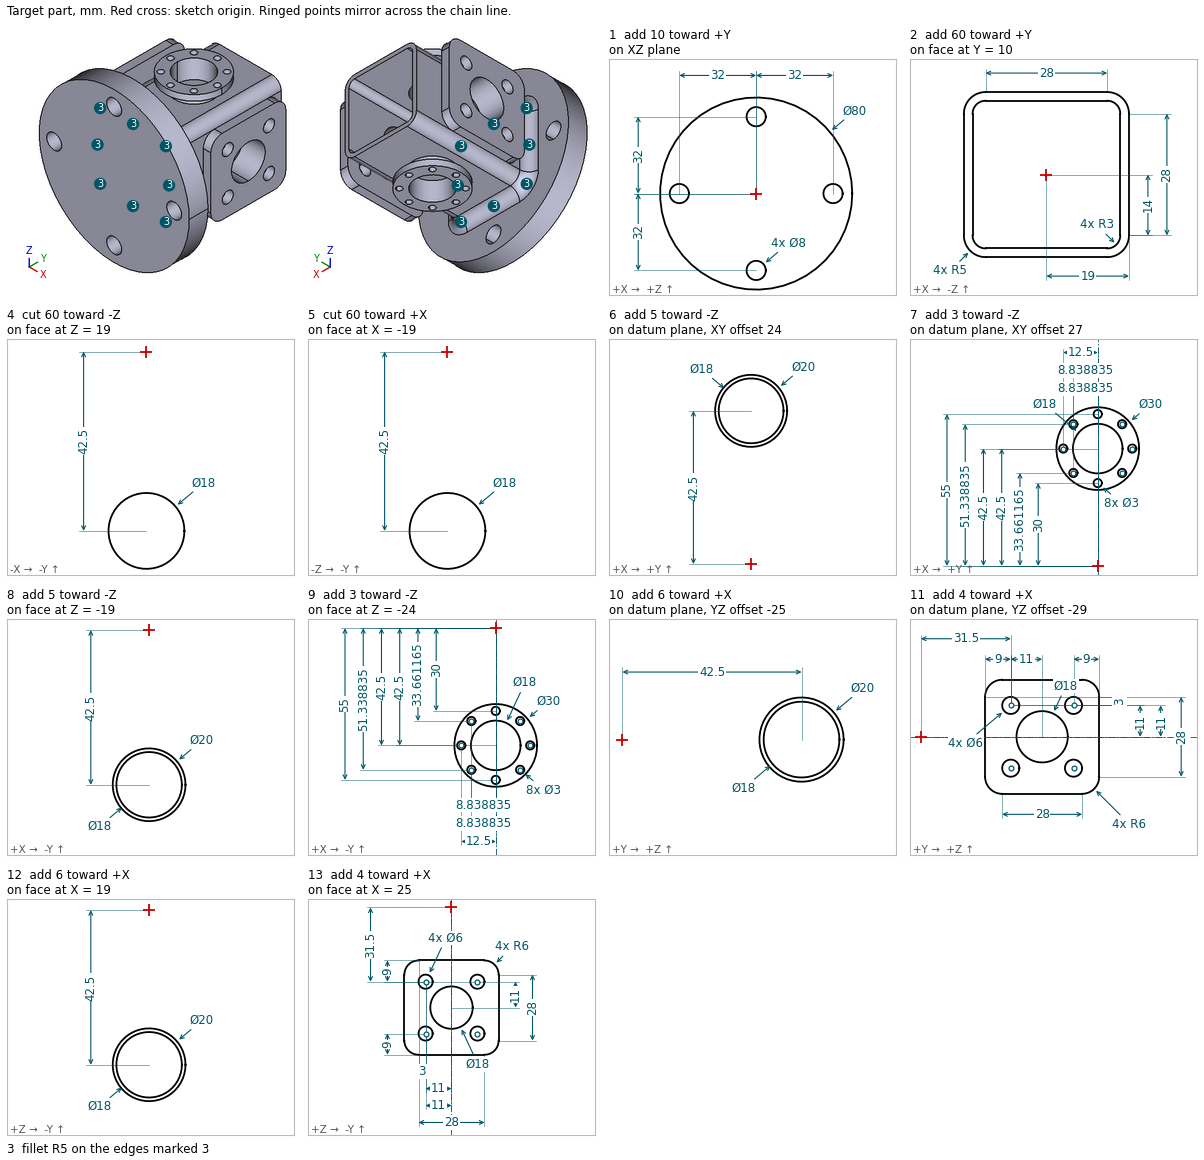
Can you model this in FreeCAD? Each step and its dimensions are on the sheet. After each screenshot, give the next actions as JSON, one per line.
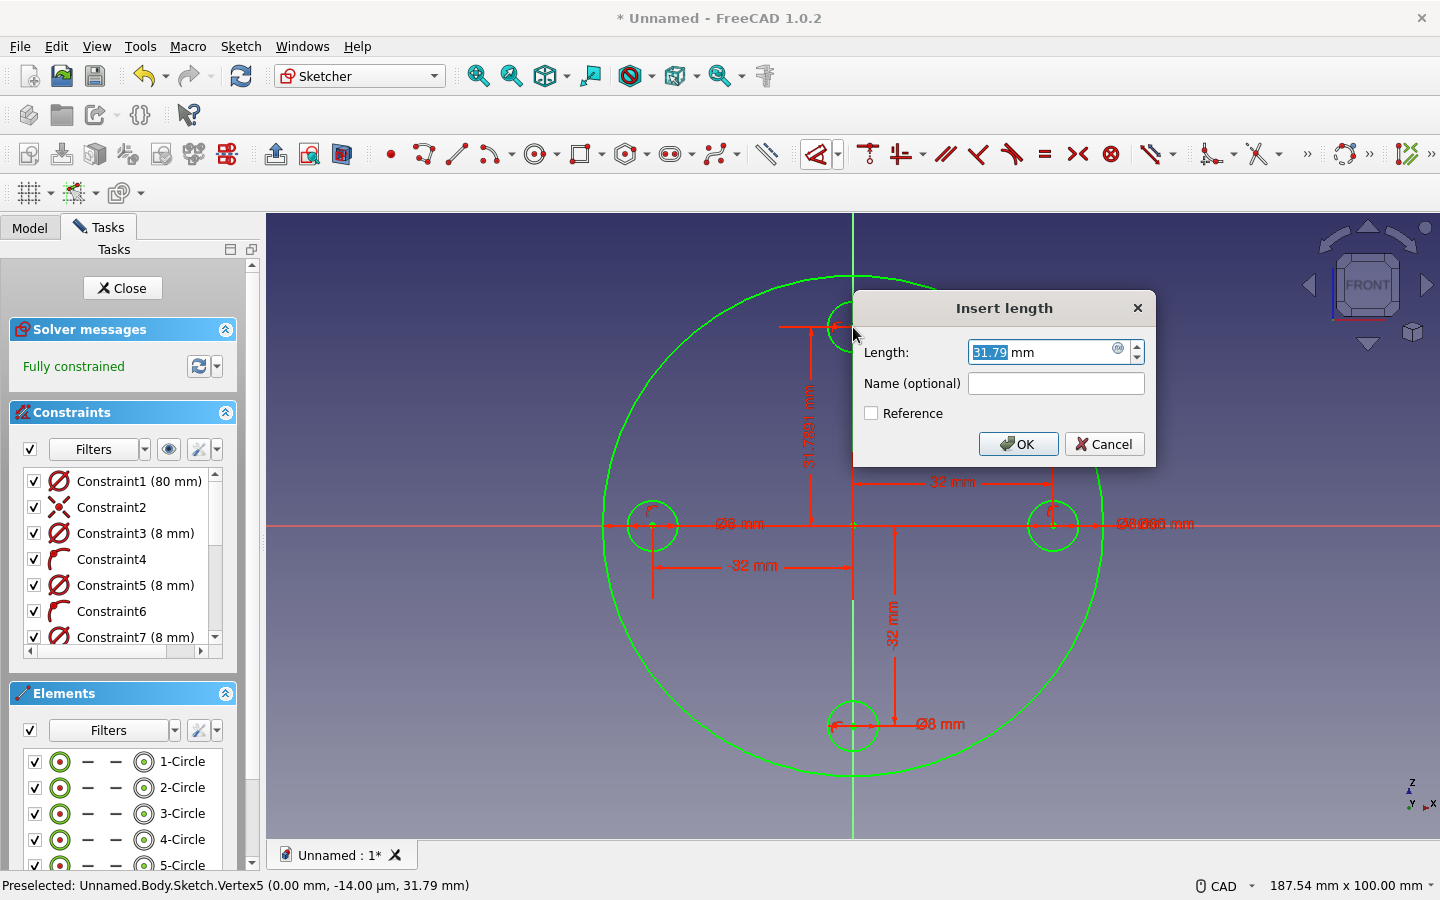
{"action": "type", "text": "32"}
{"action": "key", "text": "Return"}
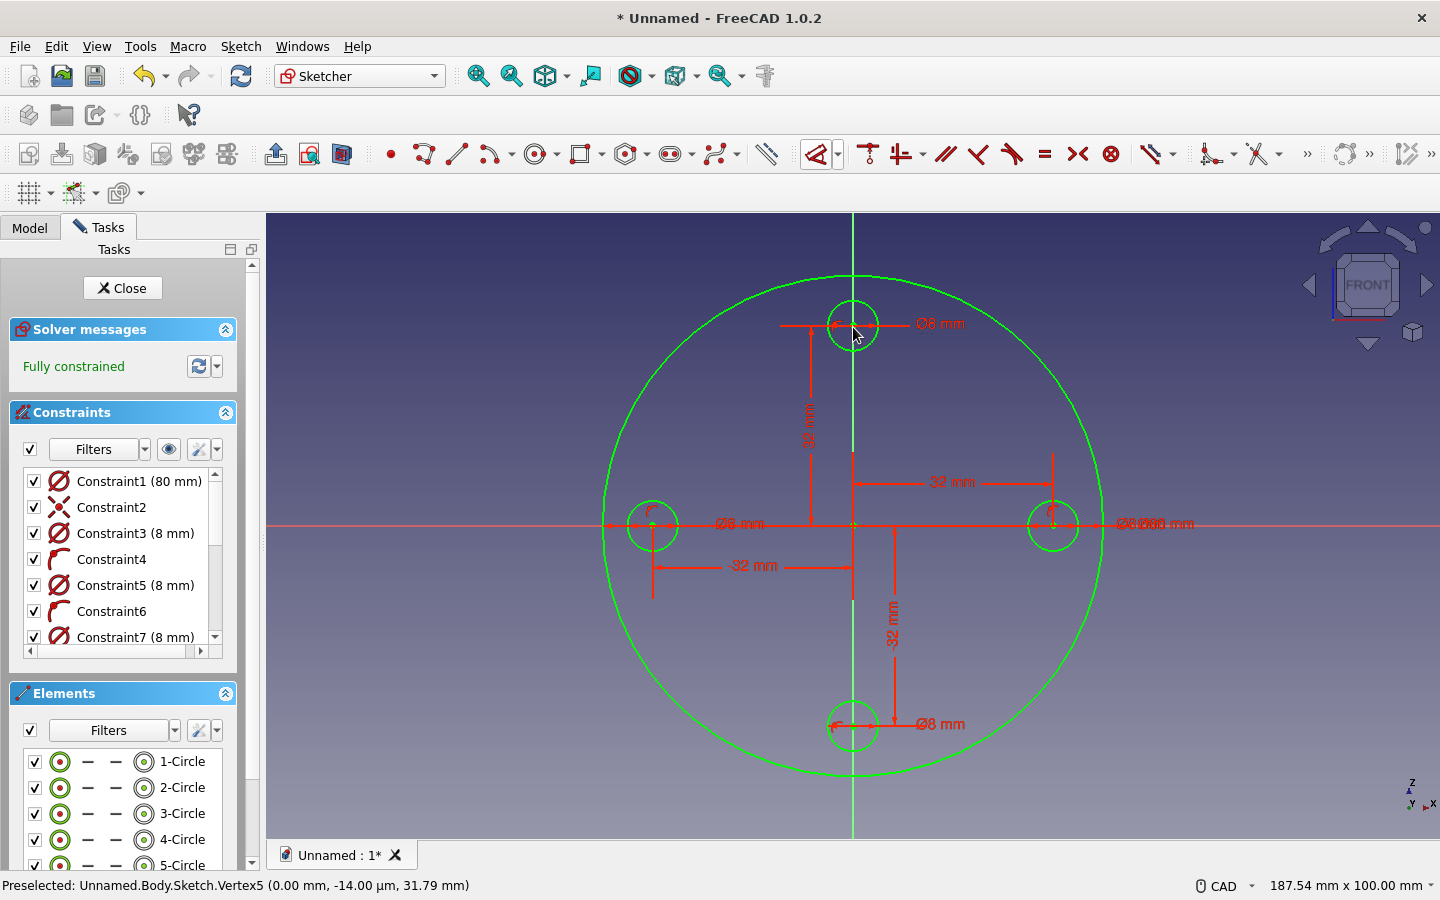
{"action": "left_click", "coordinate": [123, 288]}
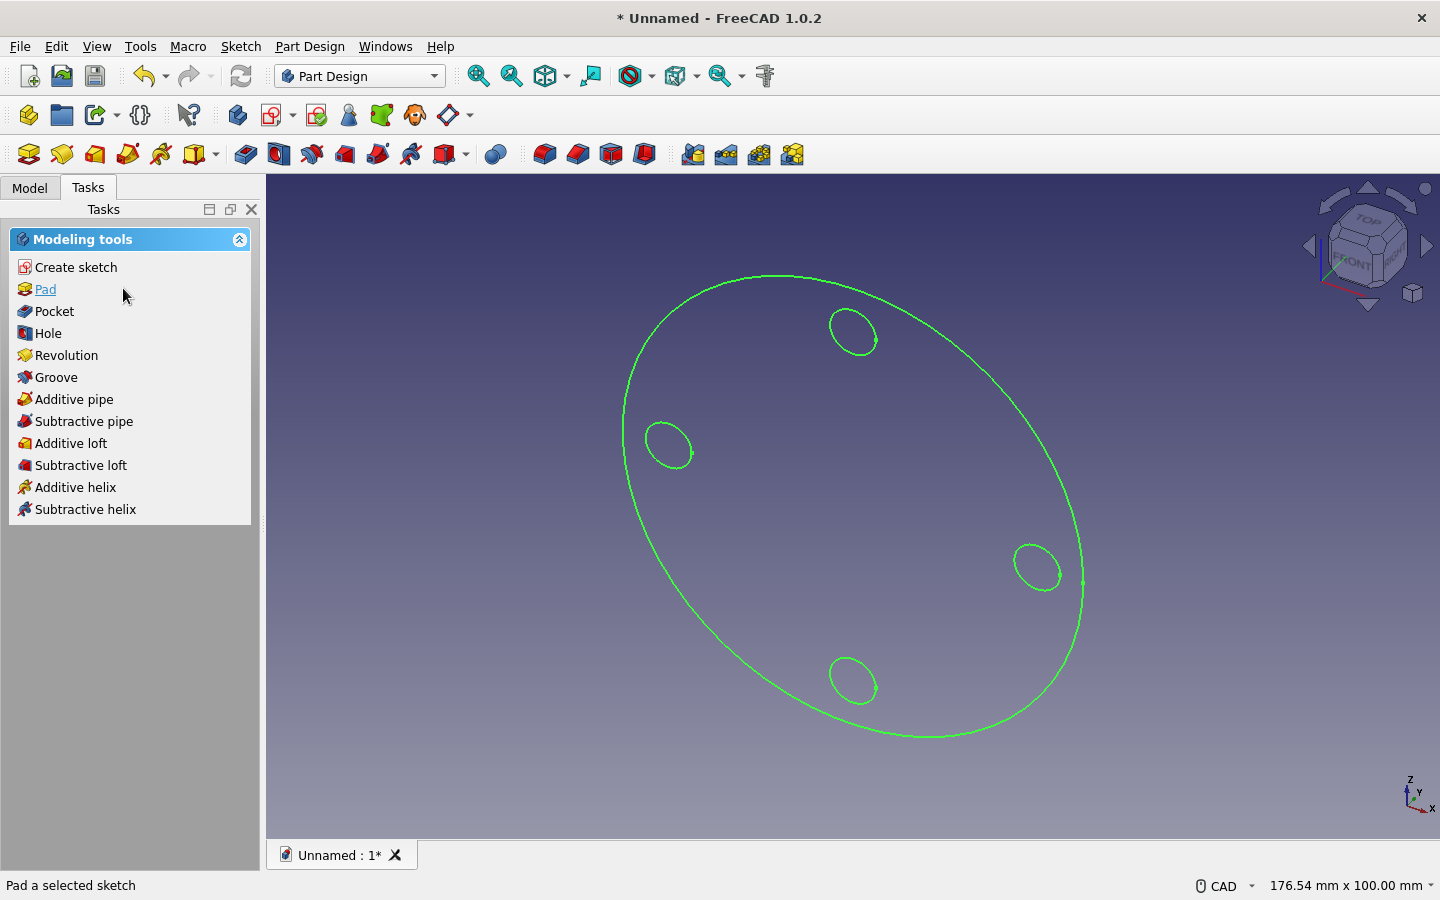
{"action": "left_click", "coordinate": [29, 154]}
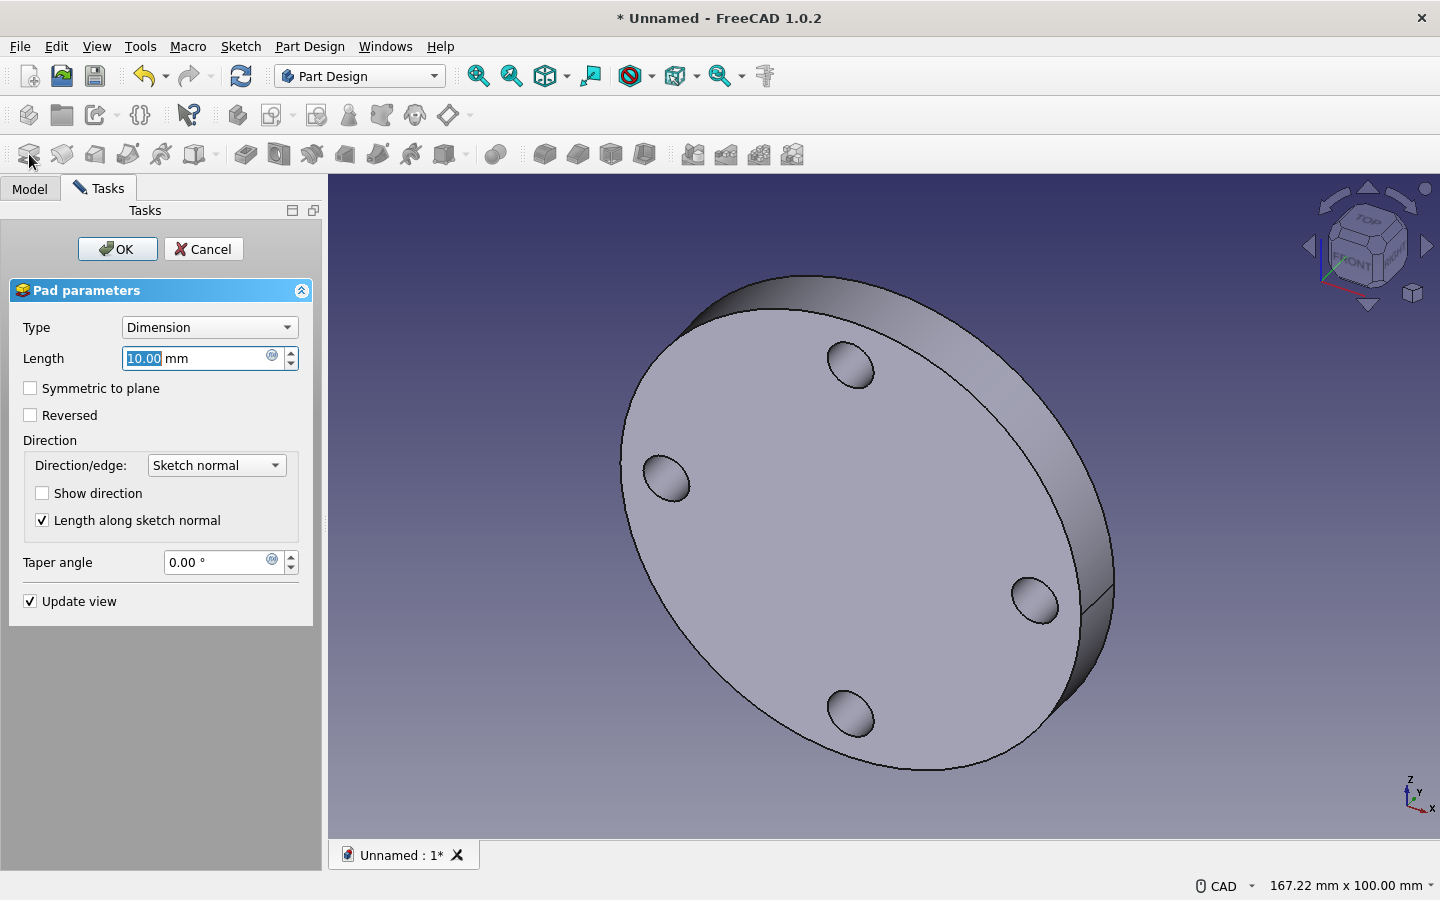
{"action": "type", "text": "10"}
{"action": "key", "text": "Tab"}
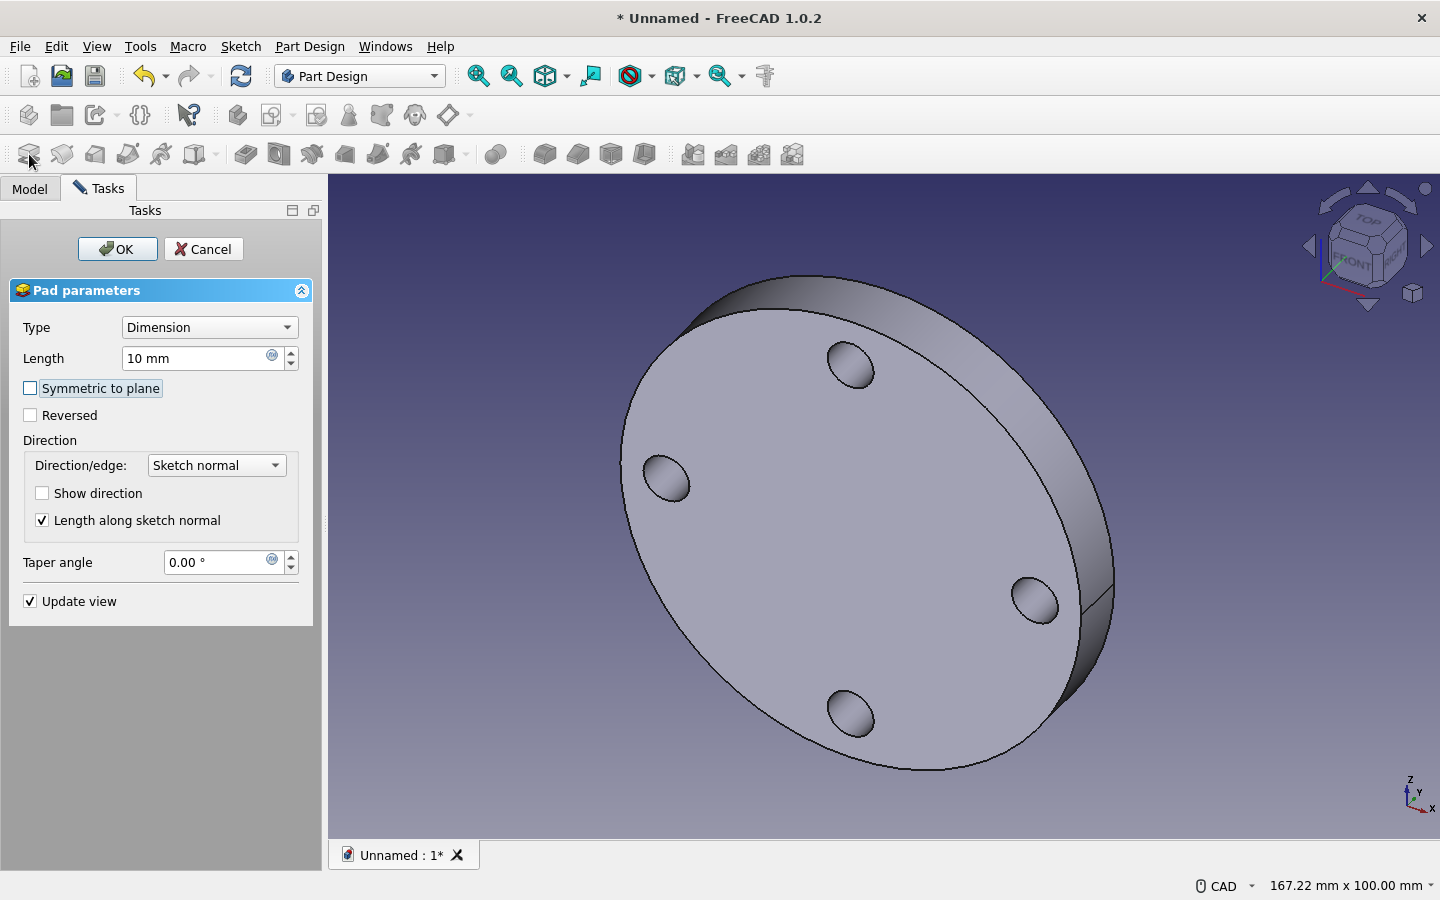
{"action": "left_click", "coordinate": [31, 415]}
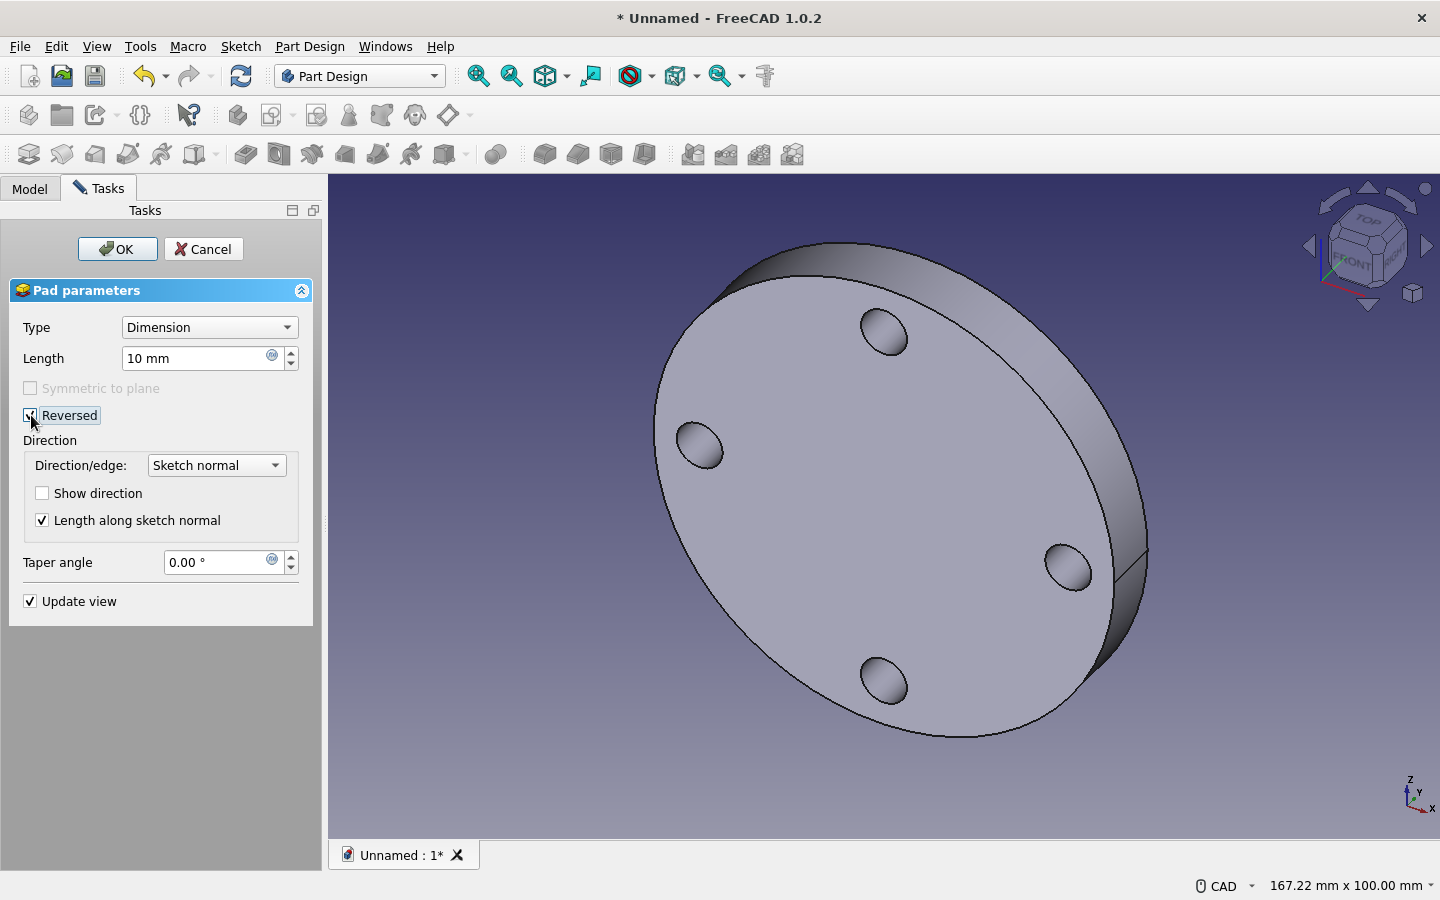
{"action": "left_click", "coordinate": [118, 249]}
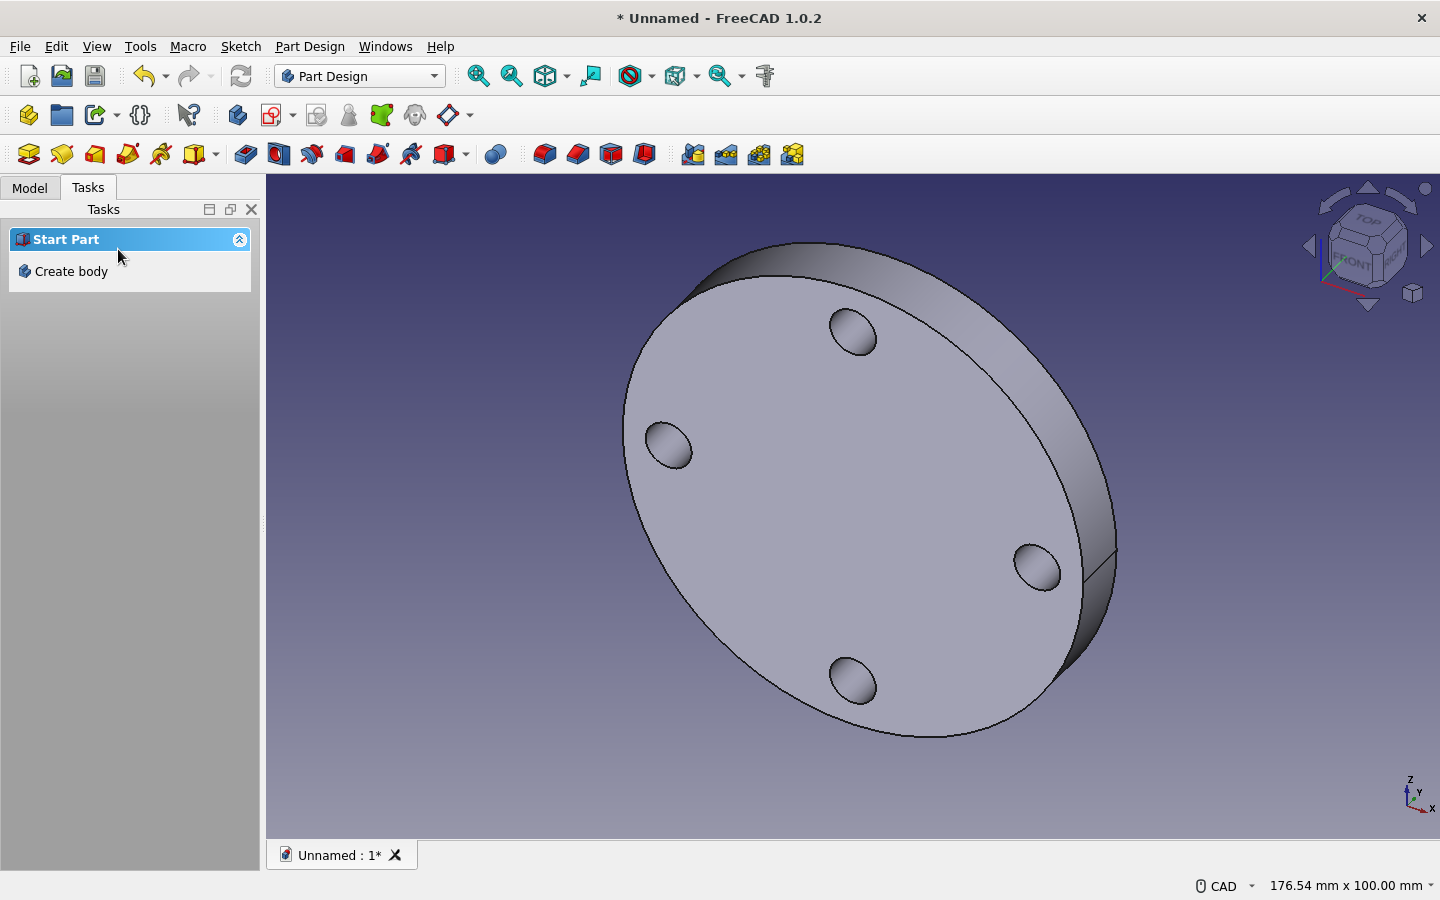
{"action": "key", "text": "4"}